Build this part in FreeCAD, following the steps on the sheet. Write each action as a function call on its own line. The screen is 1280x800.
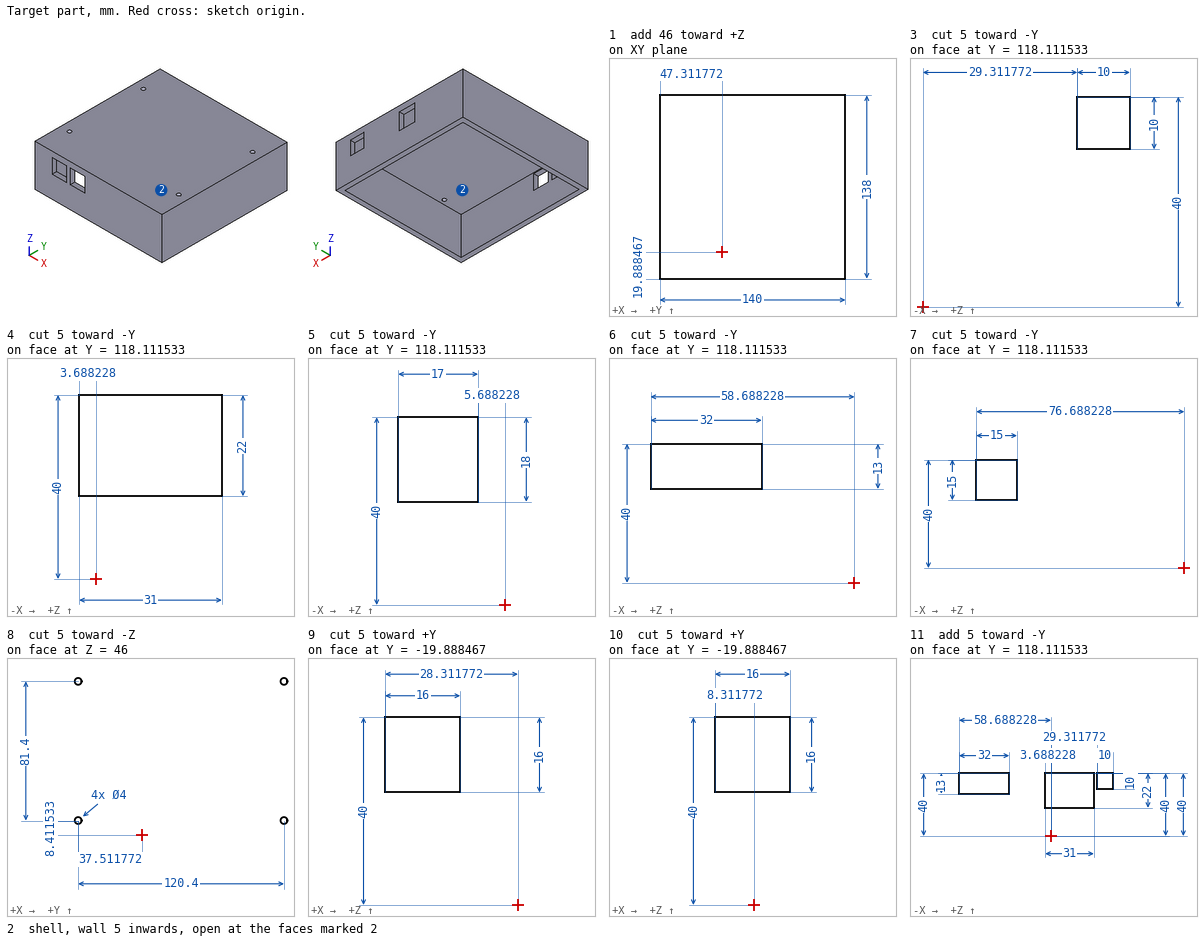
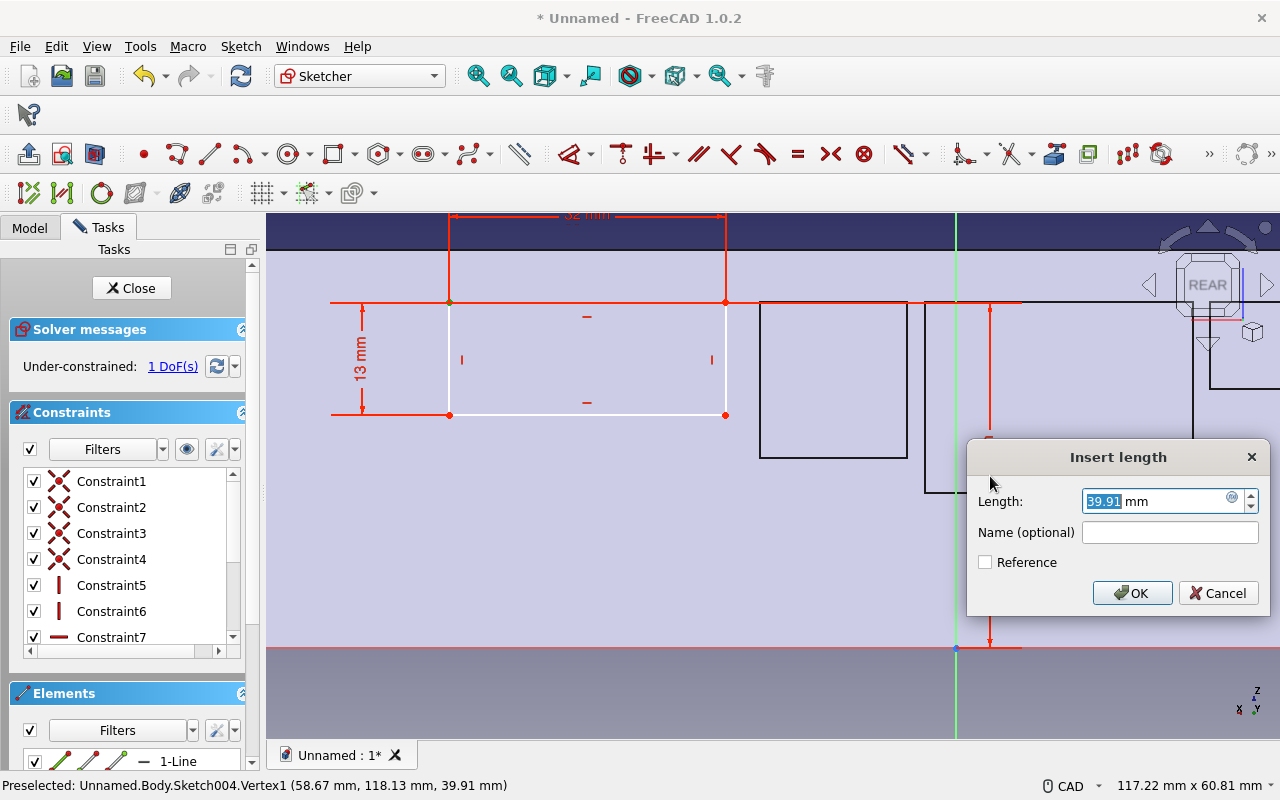
text(40)
key(Return)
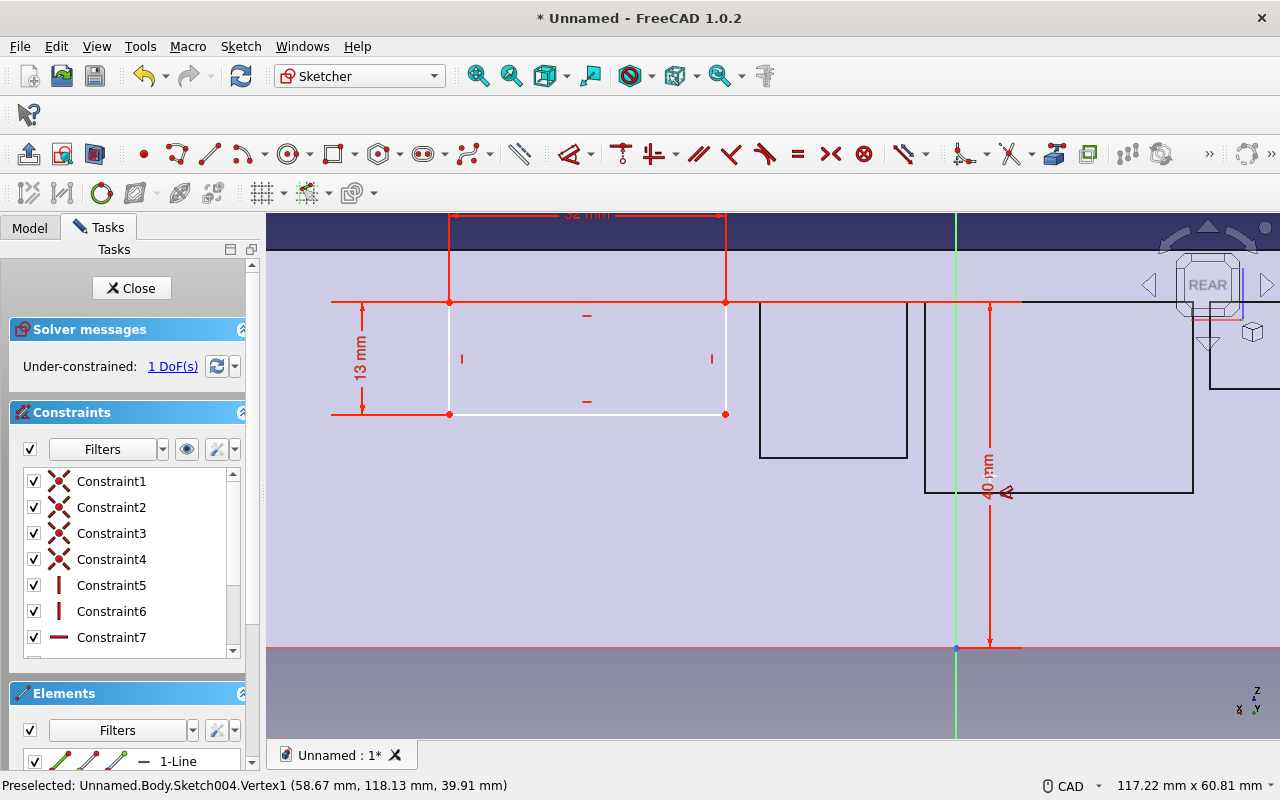
click(449, 302)
click(703, 682)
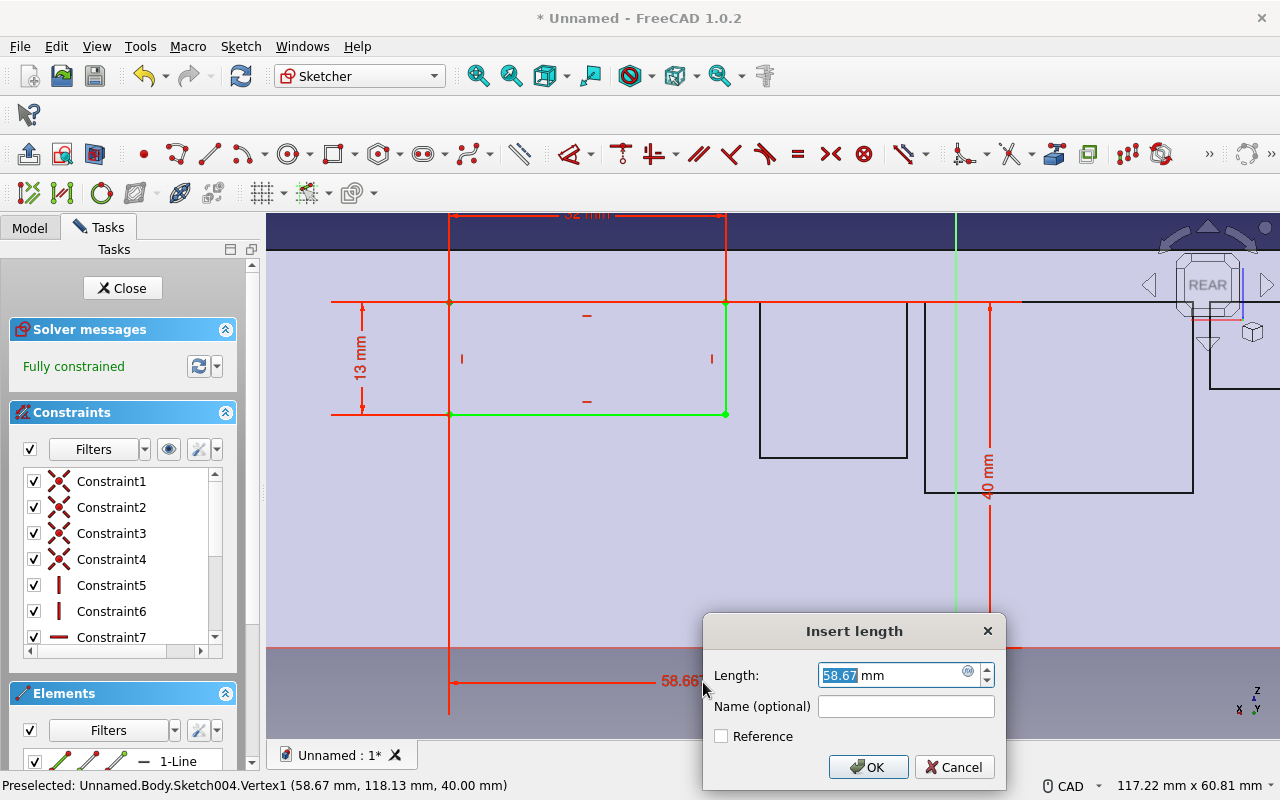
text(58.688228)
key(Return)
key(Escape)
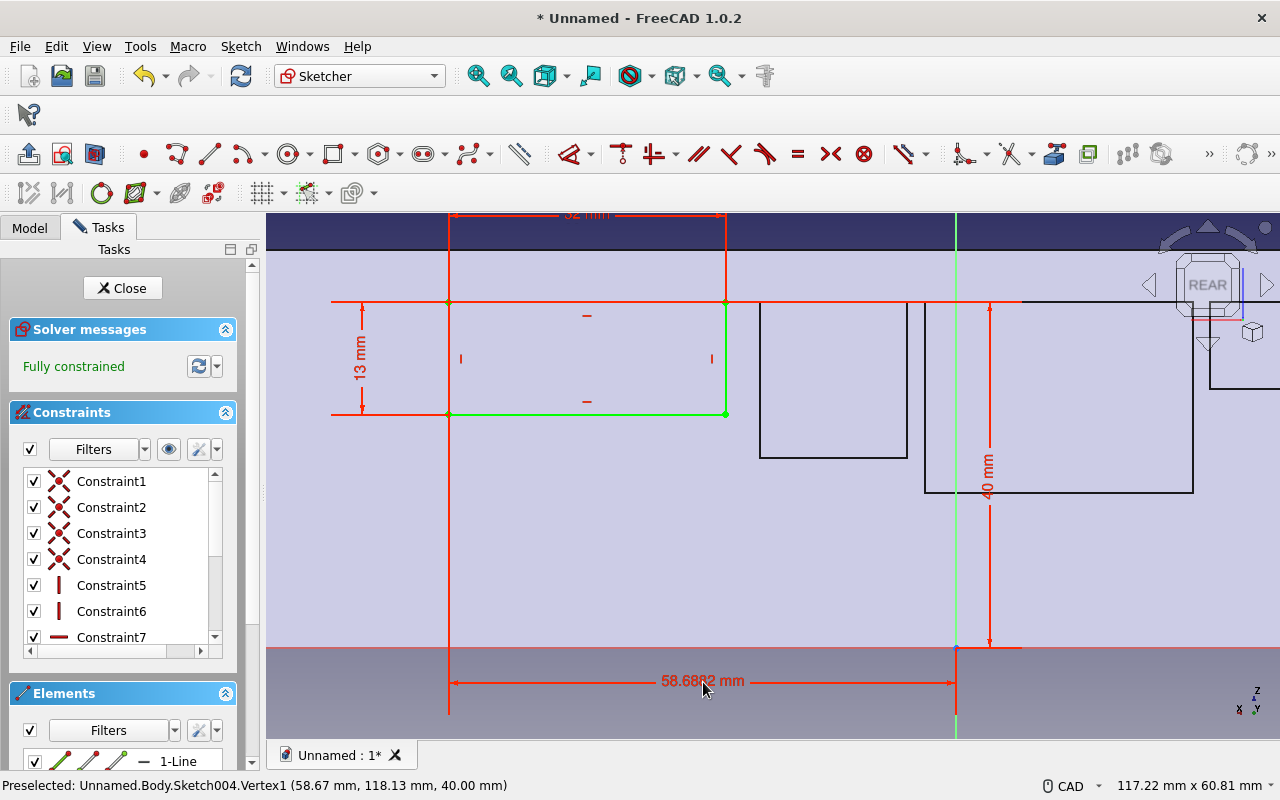
click(123, 288)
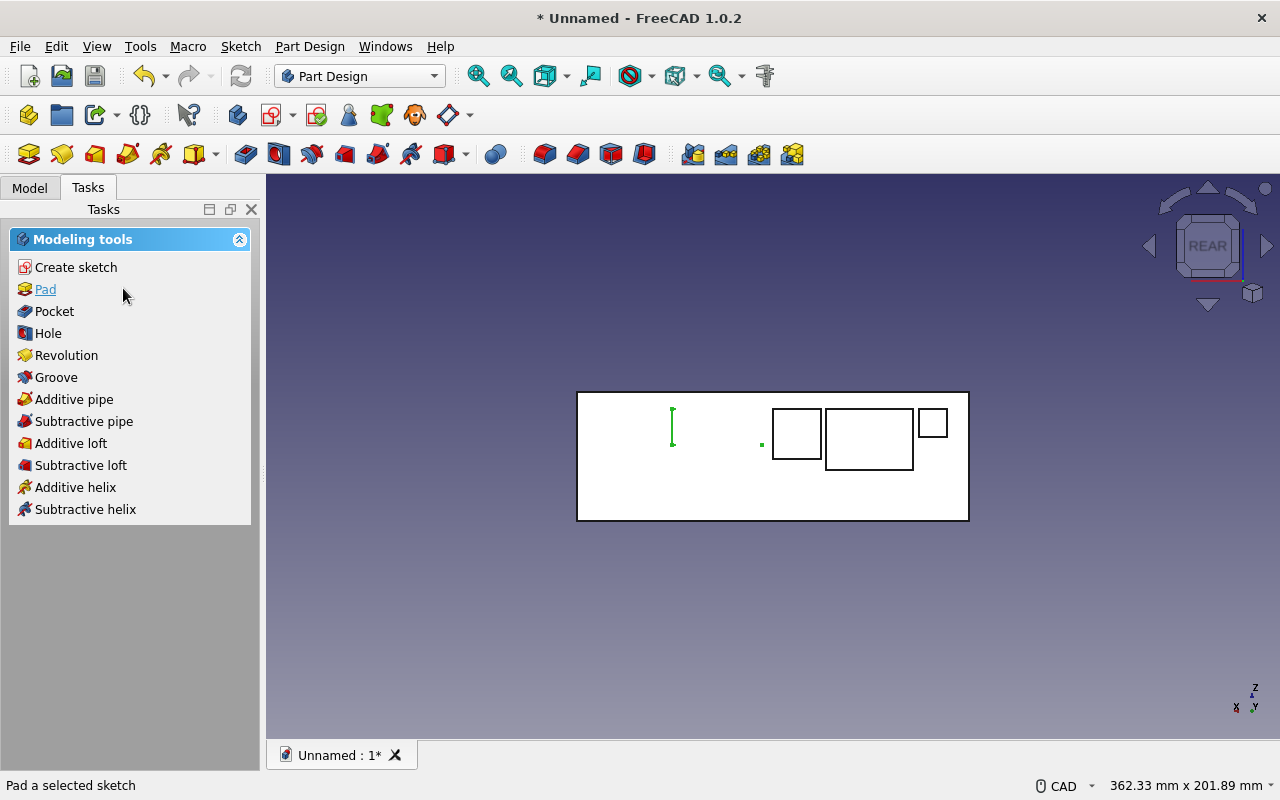
click(246, 154)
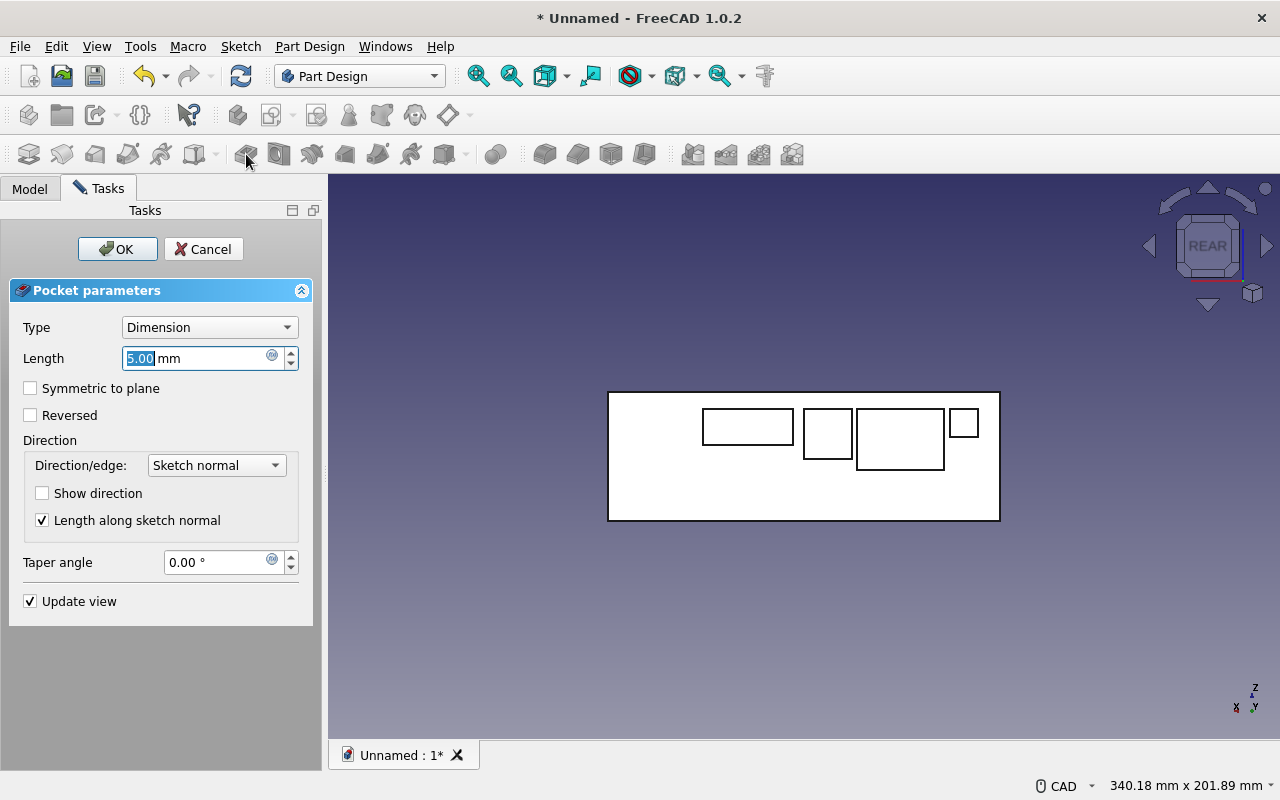
text(5)
key(Tab)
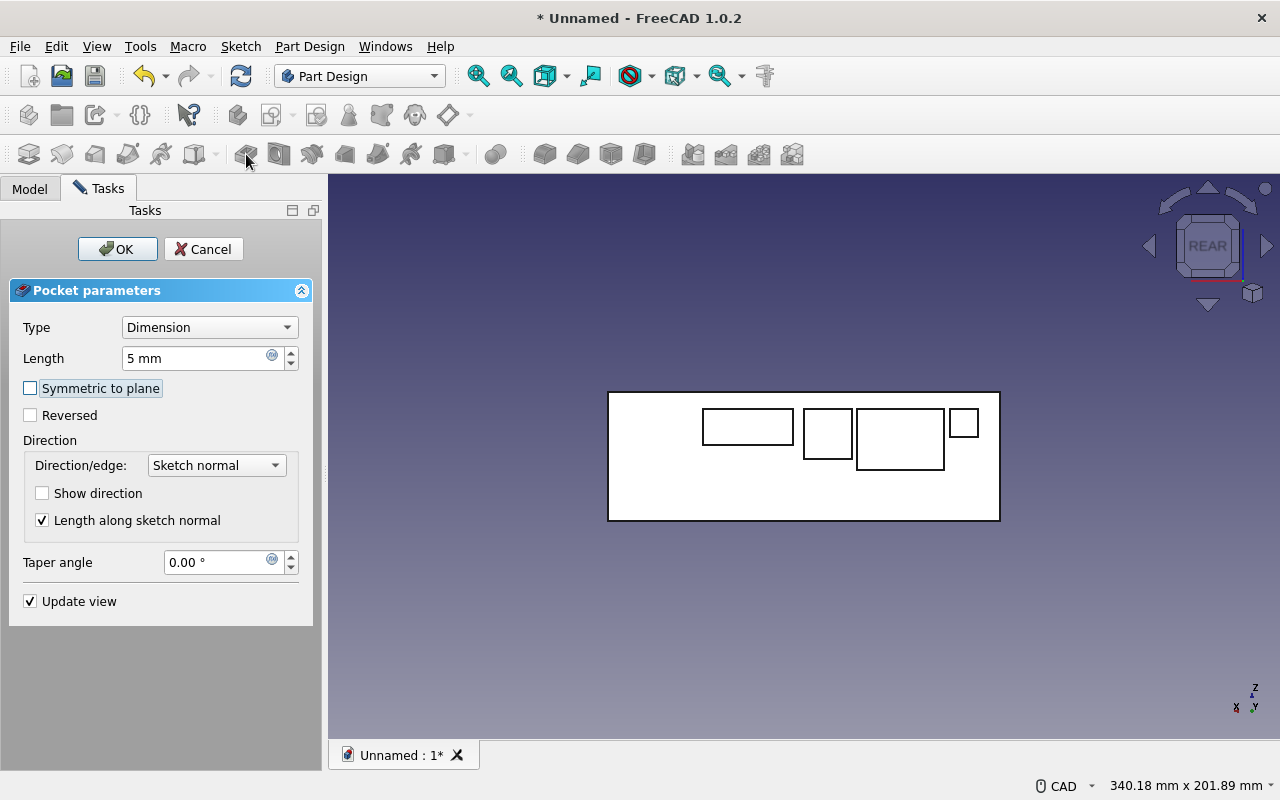
click(118, 249)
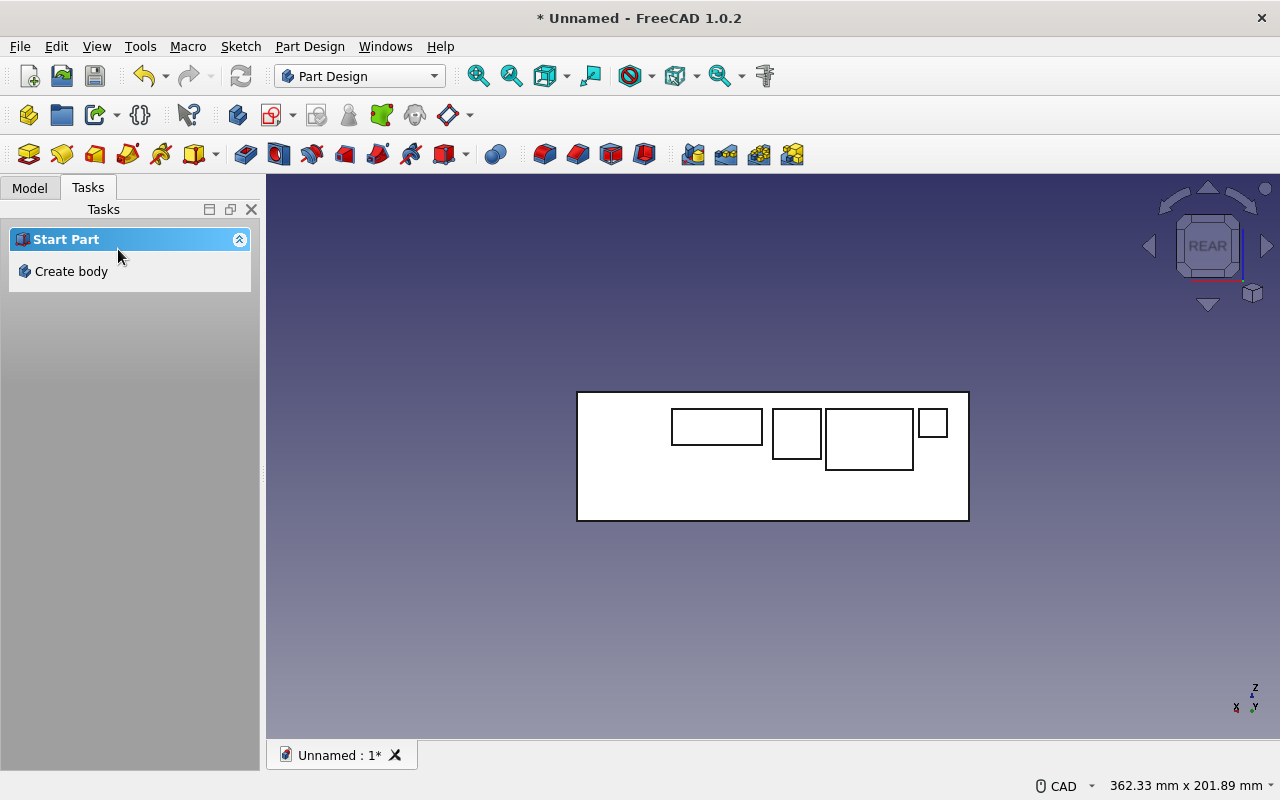
click(479, 76)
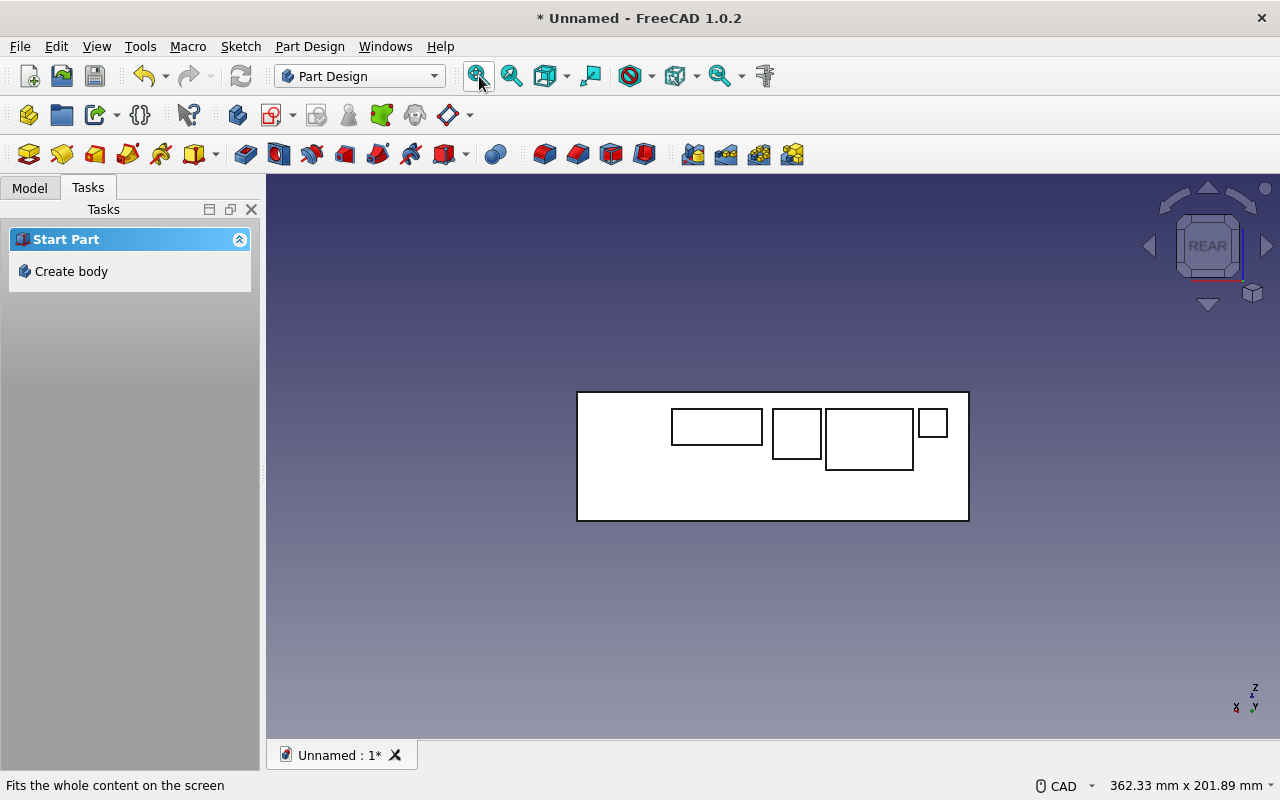
click(661, 474)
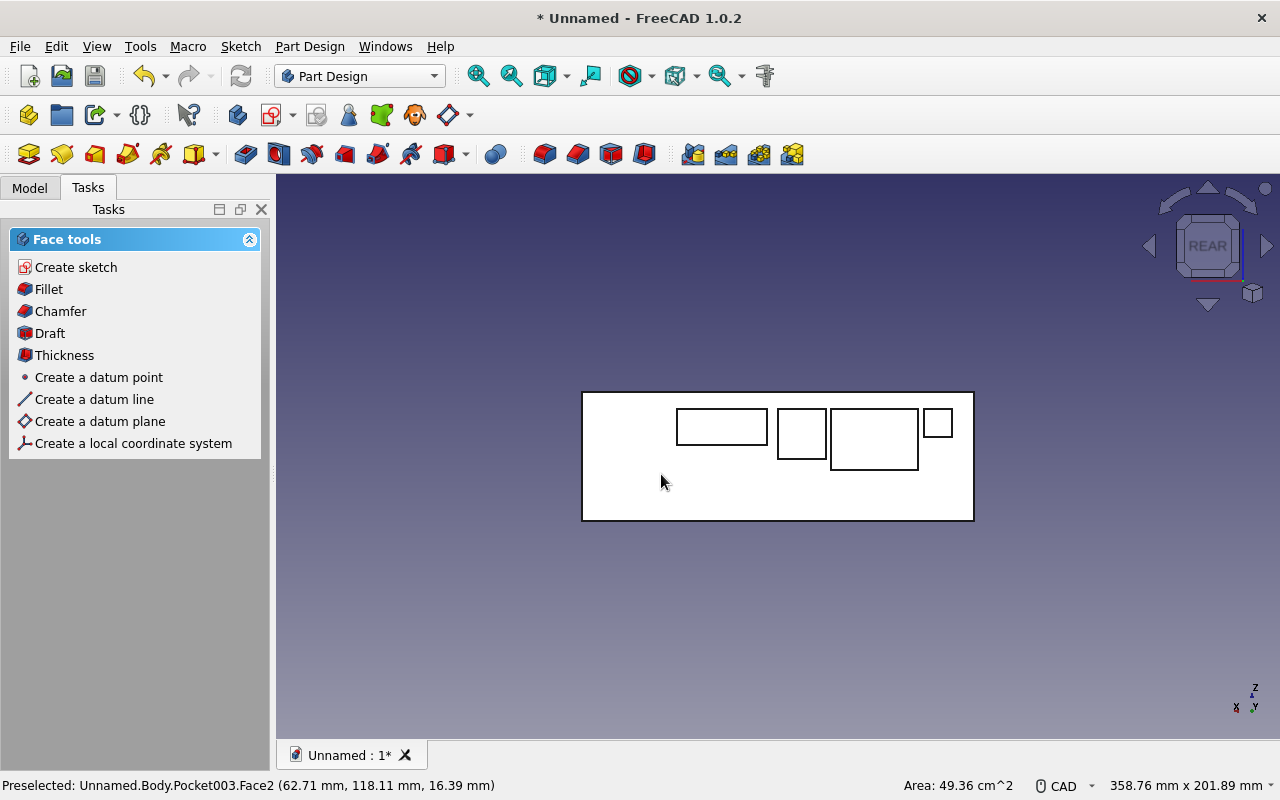
click(270, 116)